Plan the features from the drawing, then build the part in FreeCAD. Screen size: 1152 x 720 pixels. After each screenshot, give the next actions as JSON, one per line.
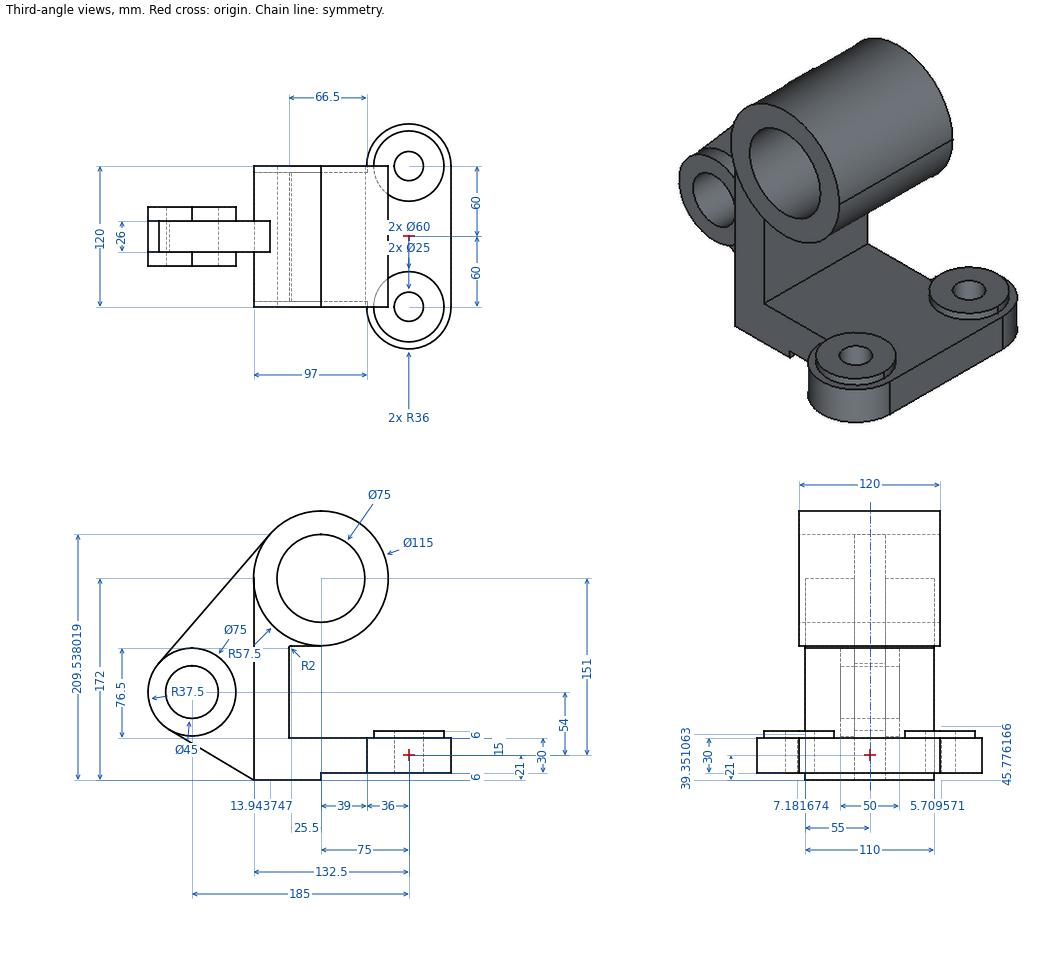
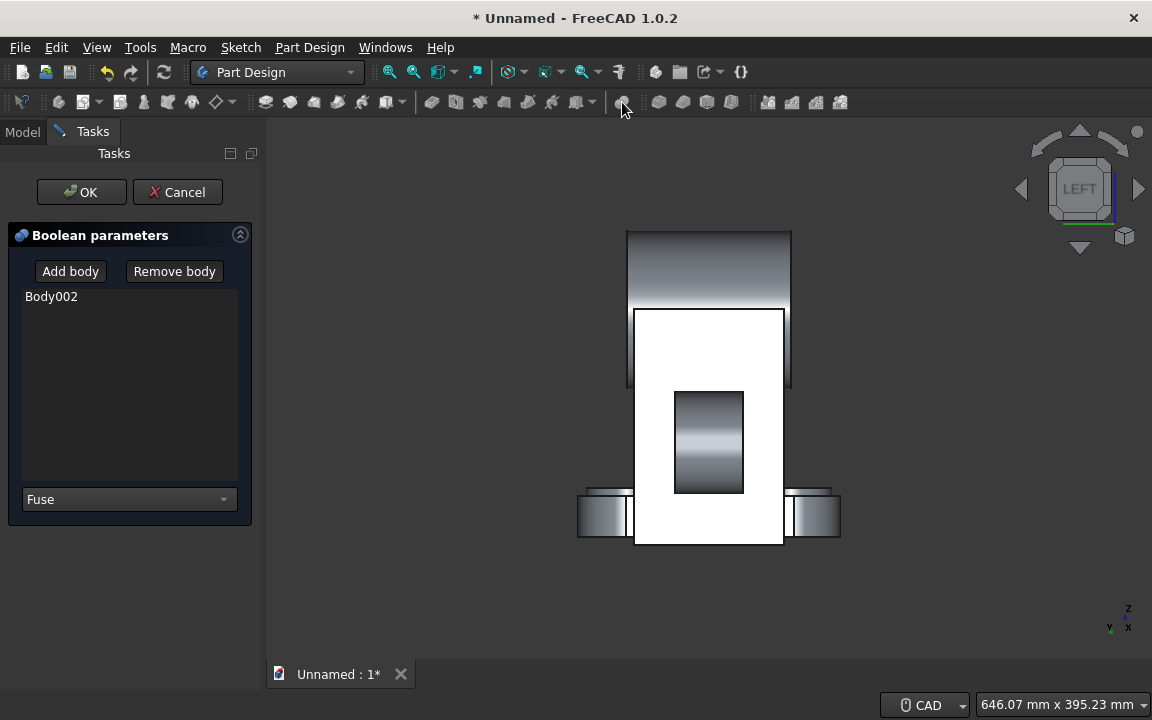
{"action": "left_click", "coordinate": [82, 192]}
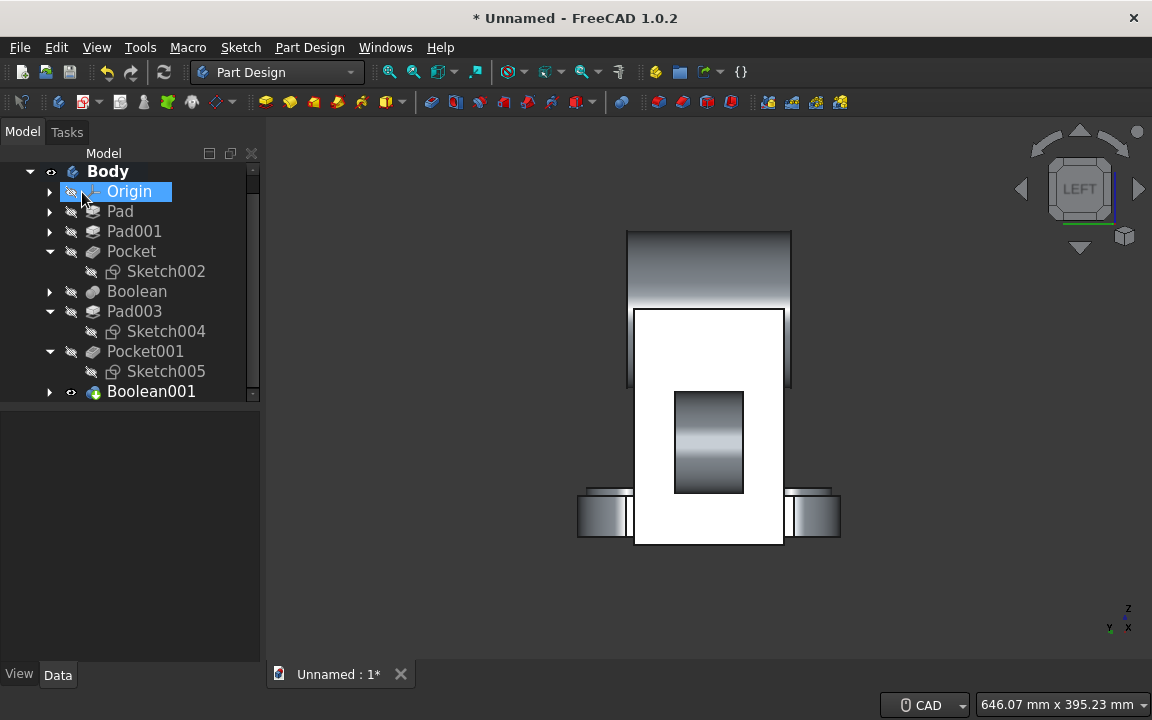
{"action": "left_click", "coordinate": [84, 102]}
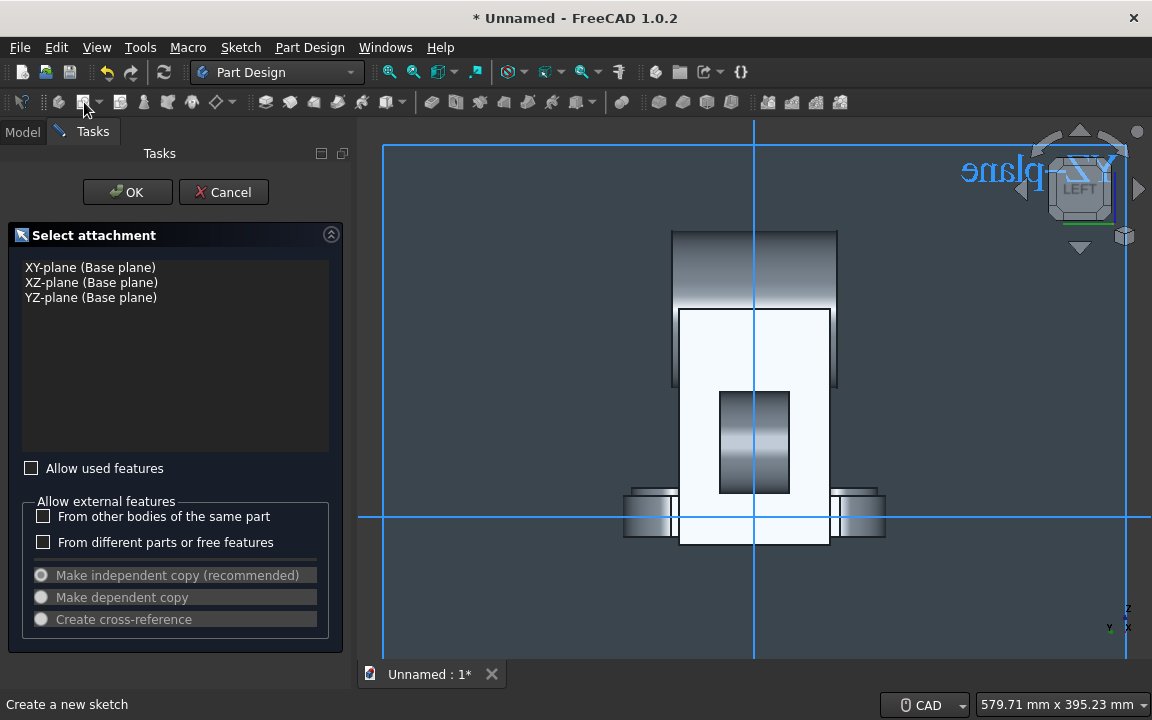
{"action": "left_click", "coordinate": [82, 282]}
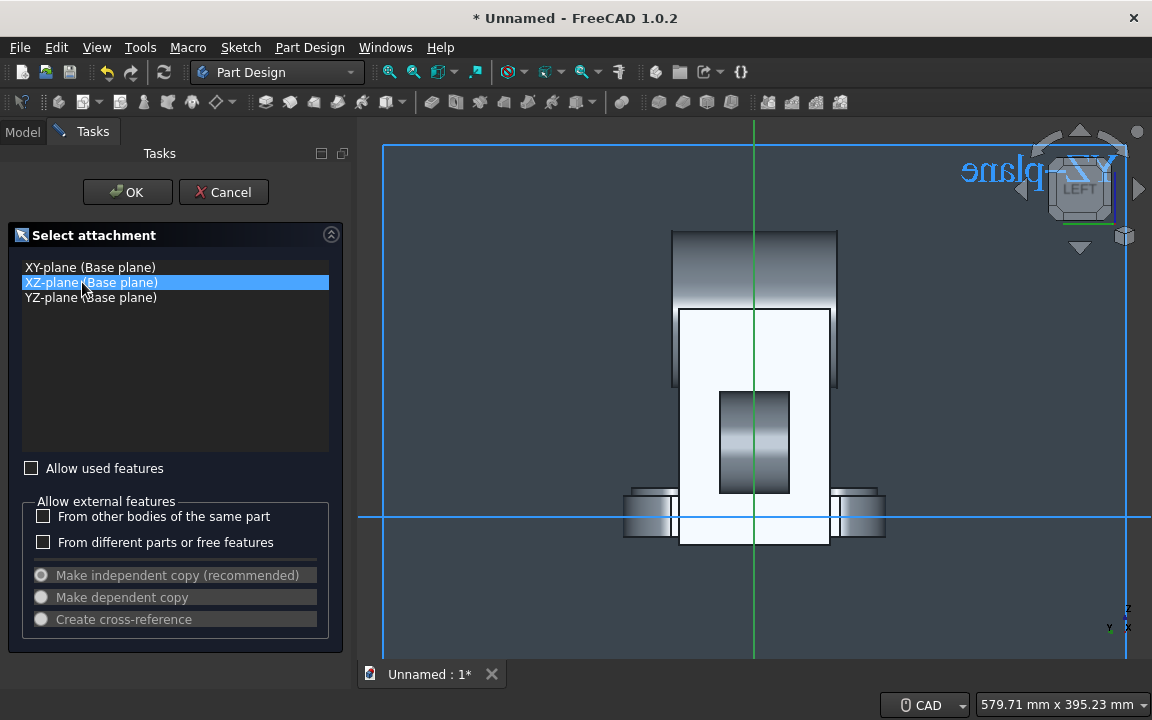
{"action": "left_click", "coordinate": [128, 192]}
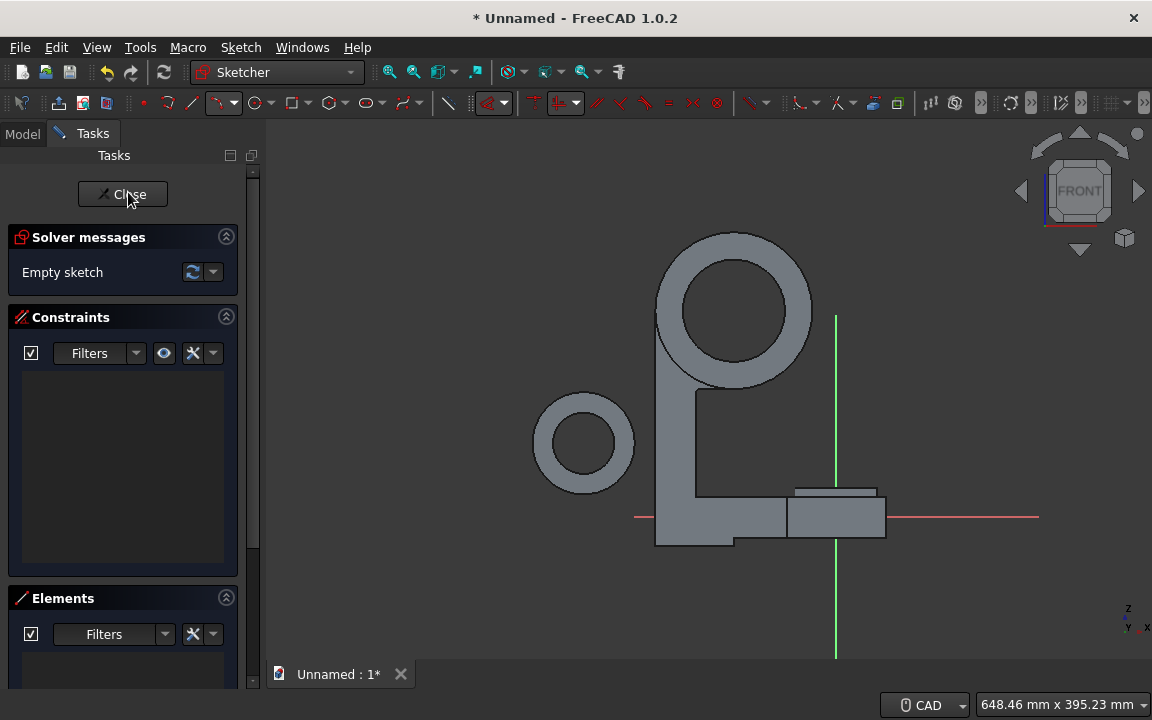
{"action": "key", "text": "q s"}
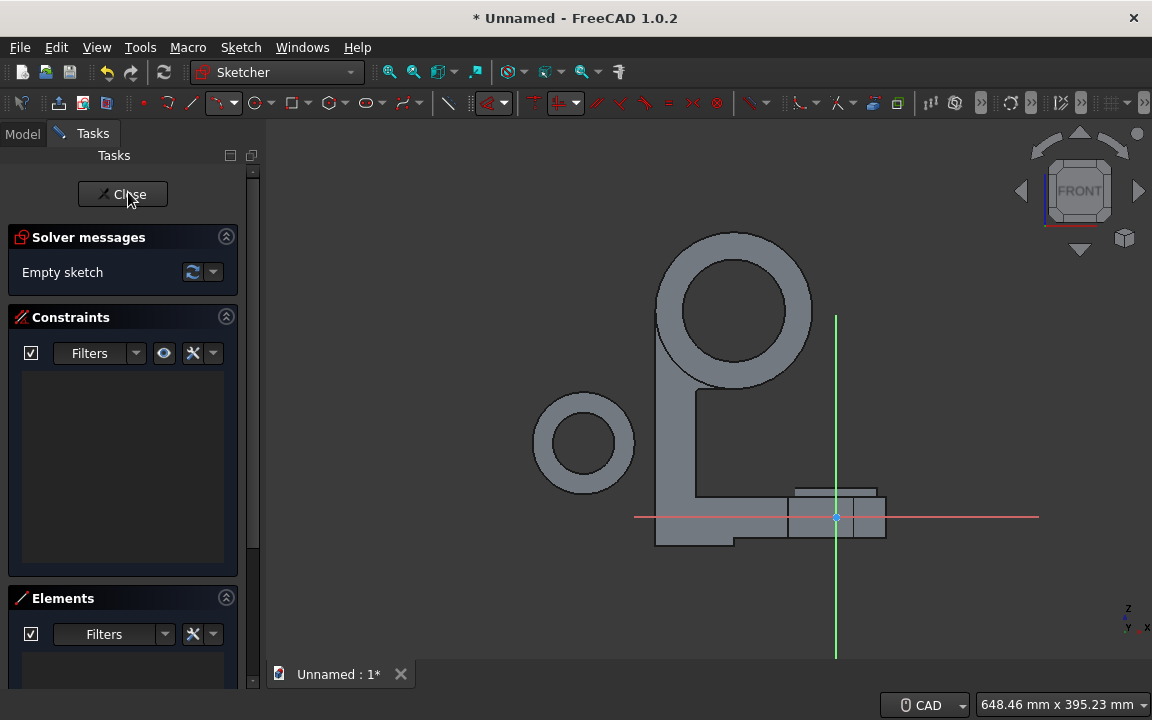
{"action": "key", "text": "g m"}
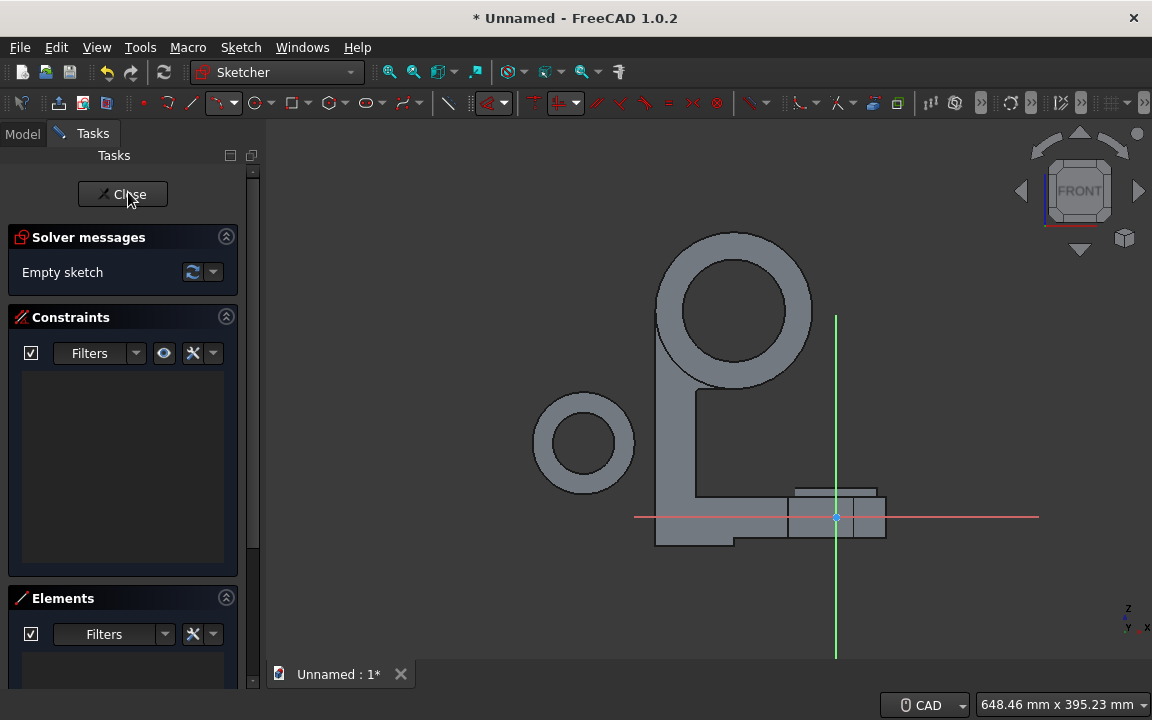
{"action": "left_click", "coordinate": [545, 410]}
{"action": "left_click", "coordinate": [674, 259]}
{"action": "left_click", "coordinate": [674, 546]}
{"action": "left_click", "coordinate": [655, 546]}
{"action": "left_click", "coordinate": [557, 487]}
{"action": "right_click", "coordinate": [557, 487]}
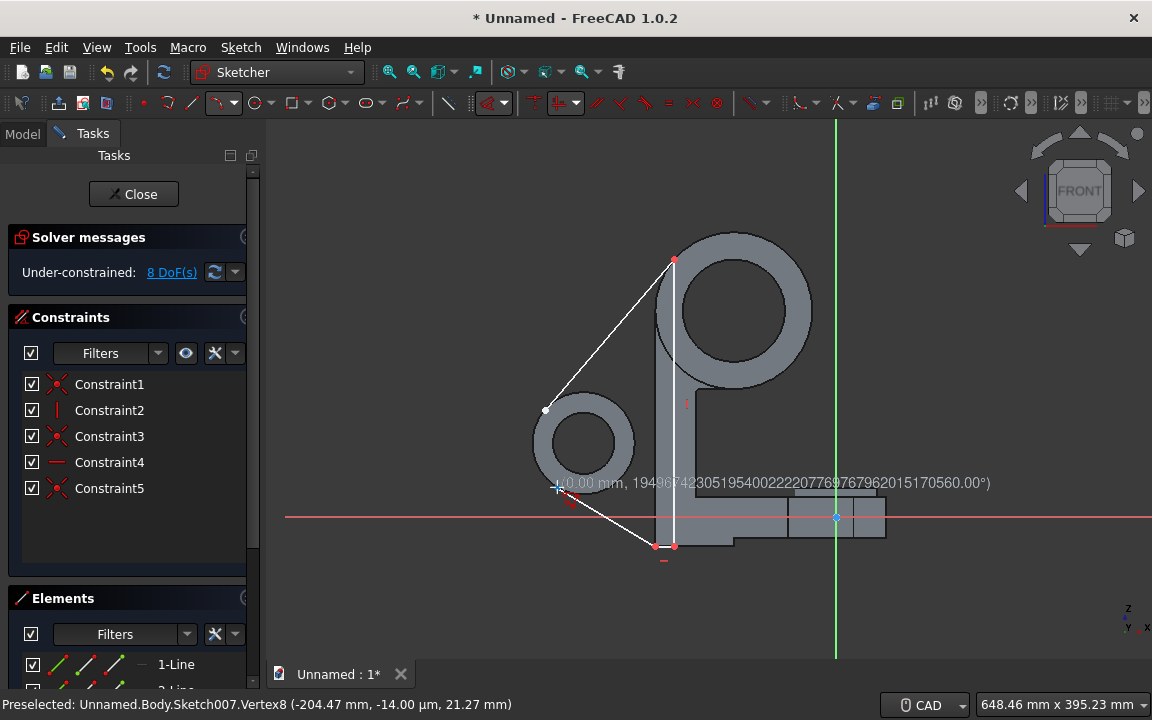
{"action": "key", "text": "g 3 a"}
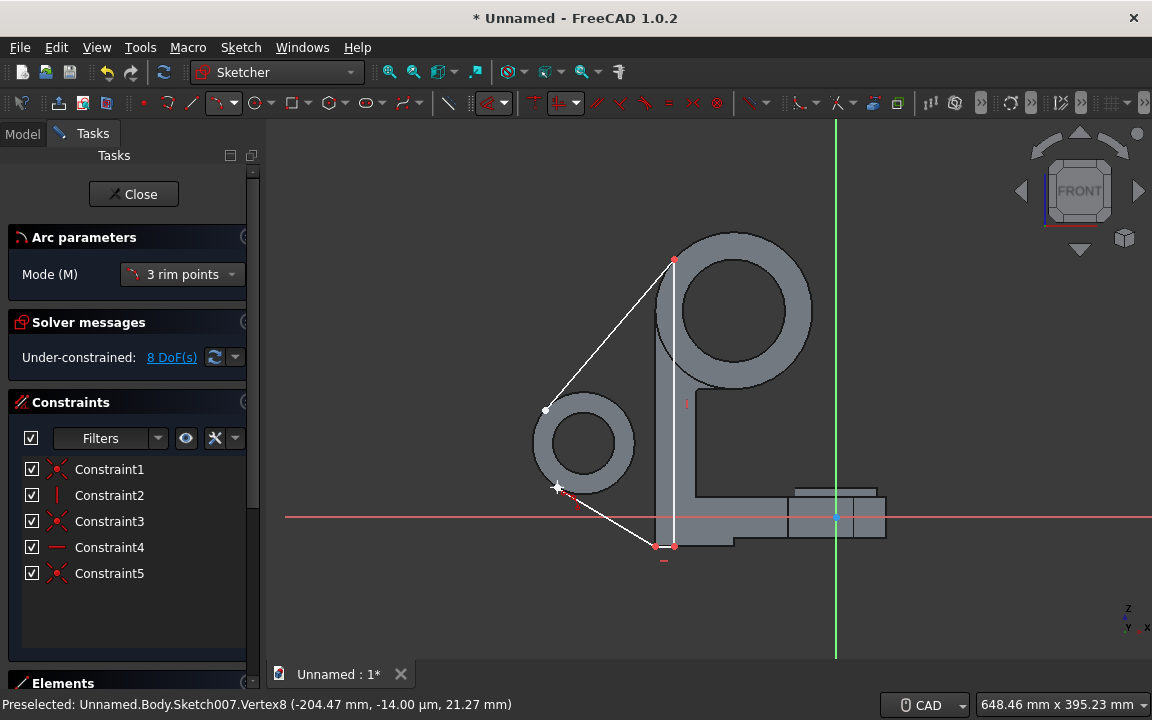
{"action": "left_click", "coordinate": [557, 488]}
{"action": "left_click", "coordinate": [545, 411]}
{"action": "left_click", "coordinate": [533, 451]}
{"action": "key", "text": "Escape"}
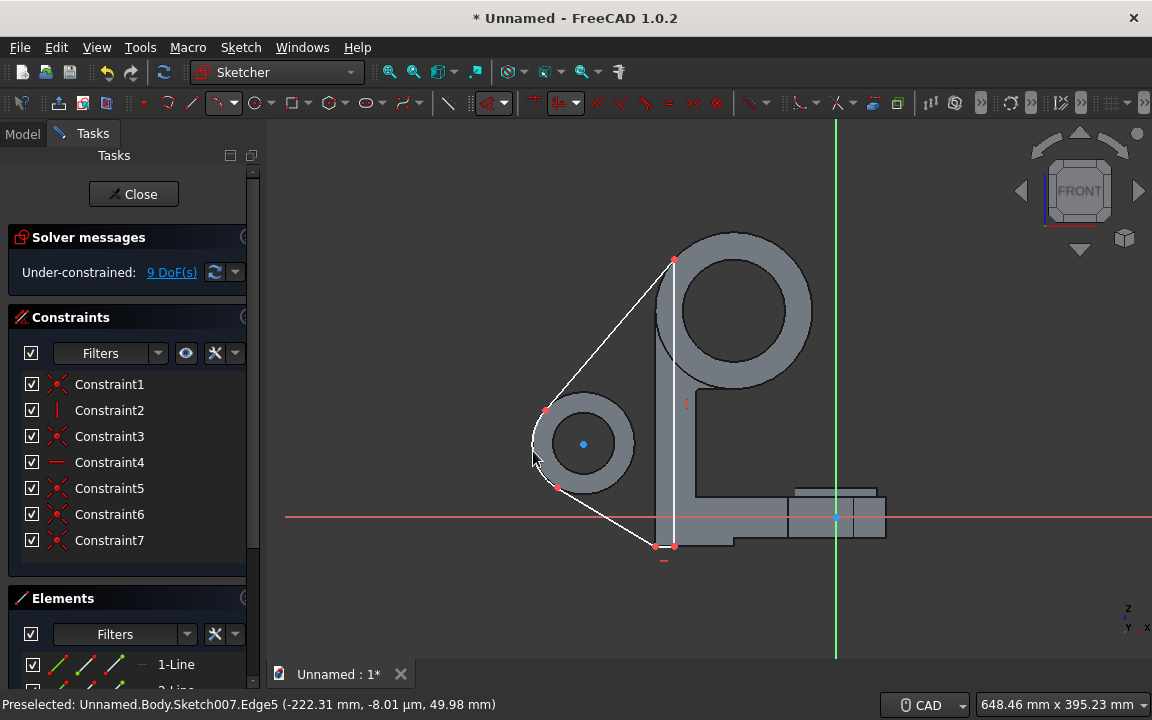
{"action": "left_click", "coordinate": [584, 366]}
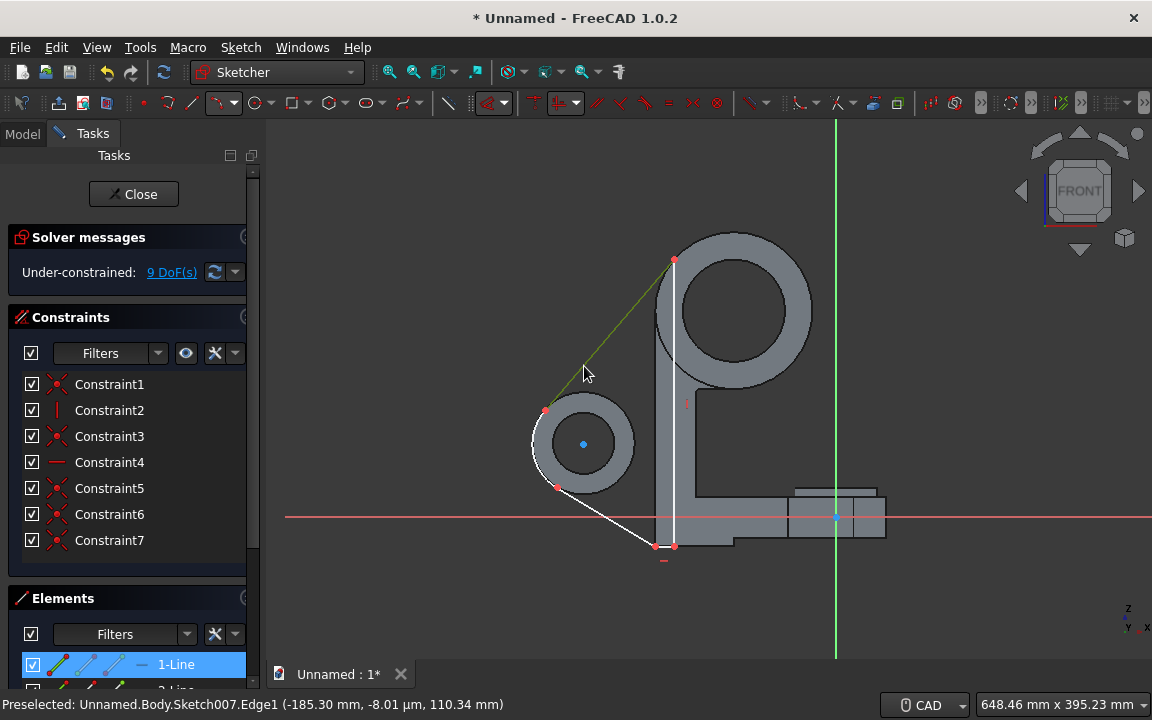
{"action": "left_click", "coordinate": [533, 435]}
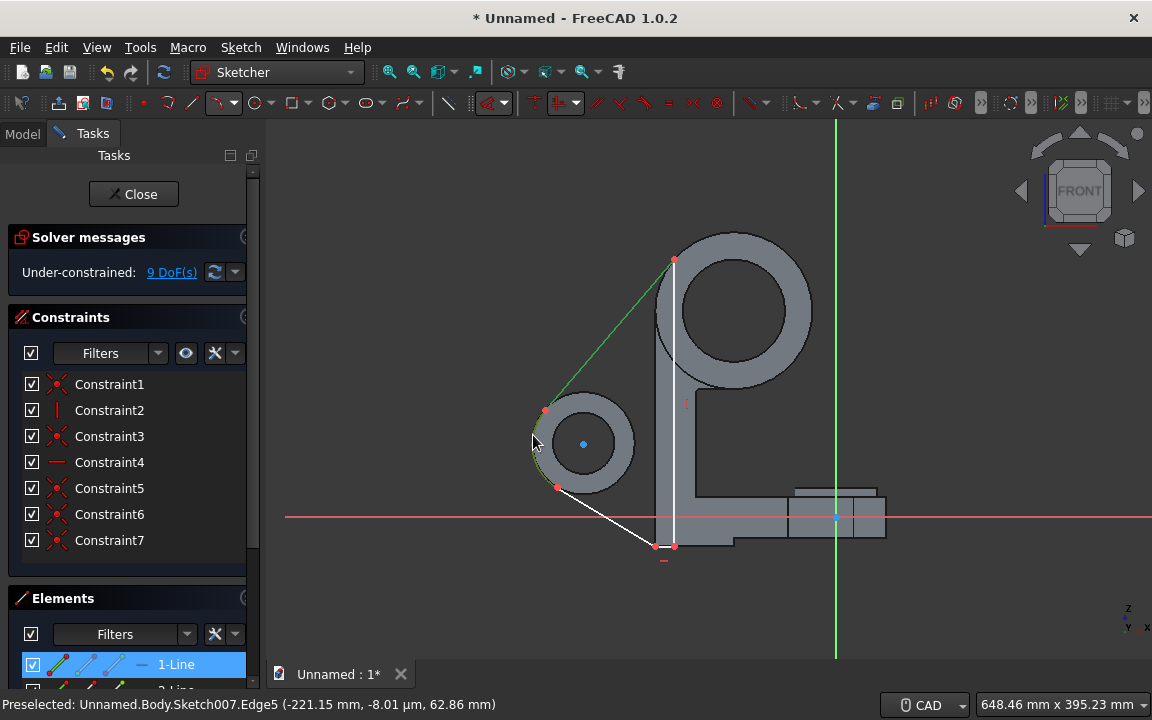
{"action": "key", "text": "t"}